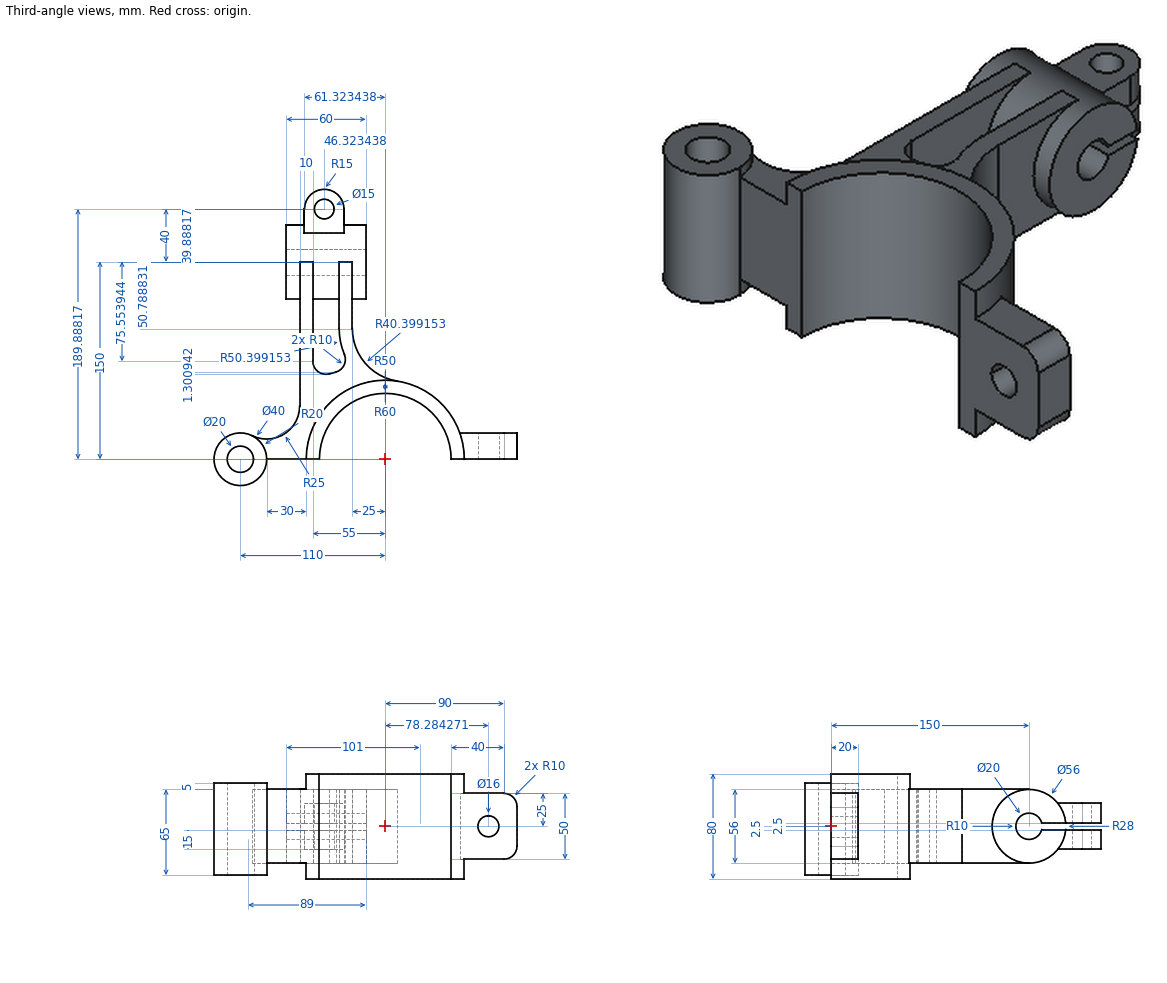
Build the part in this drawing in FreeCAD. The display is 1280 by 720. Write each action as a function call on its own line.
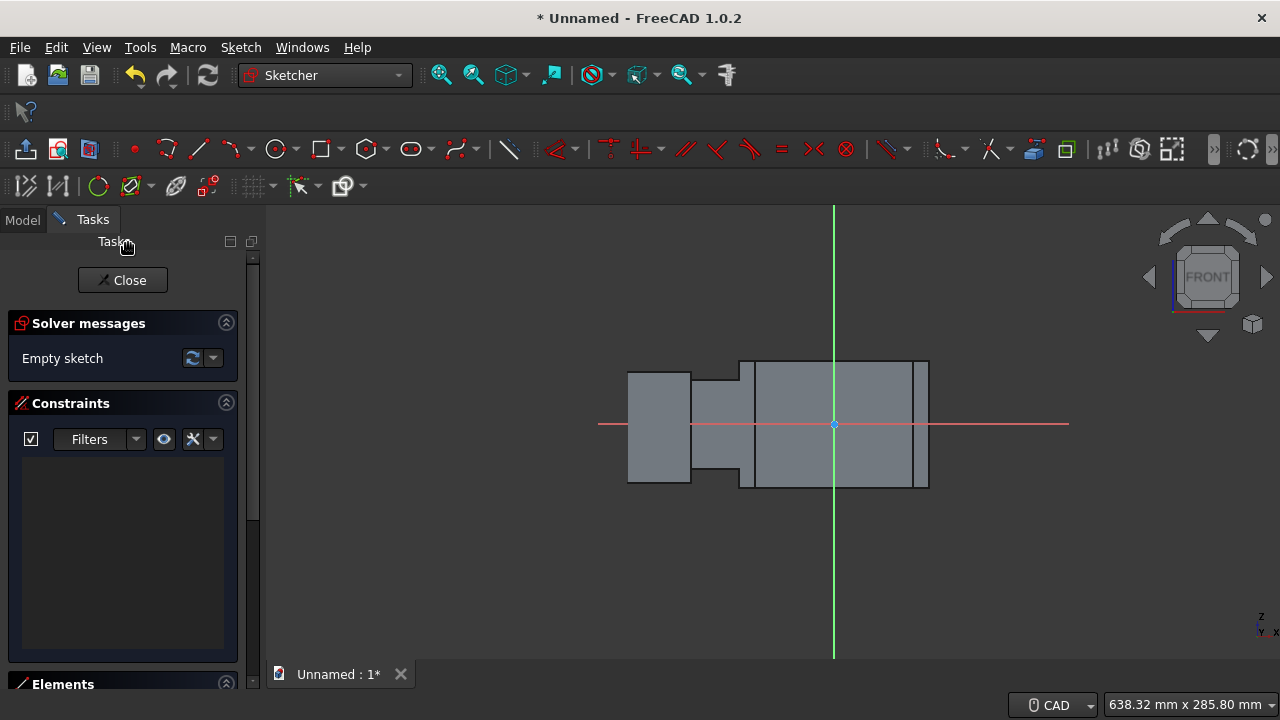
key(q)
key(s)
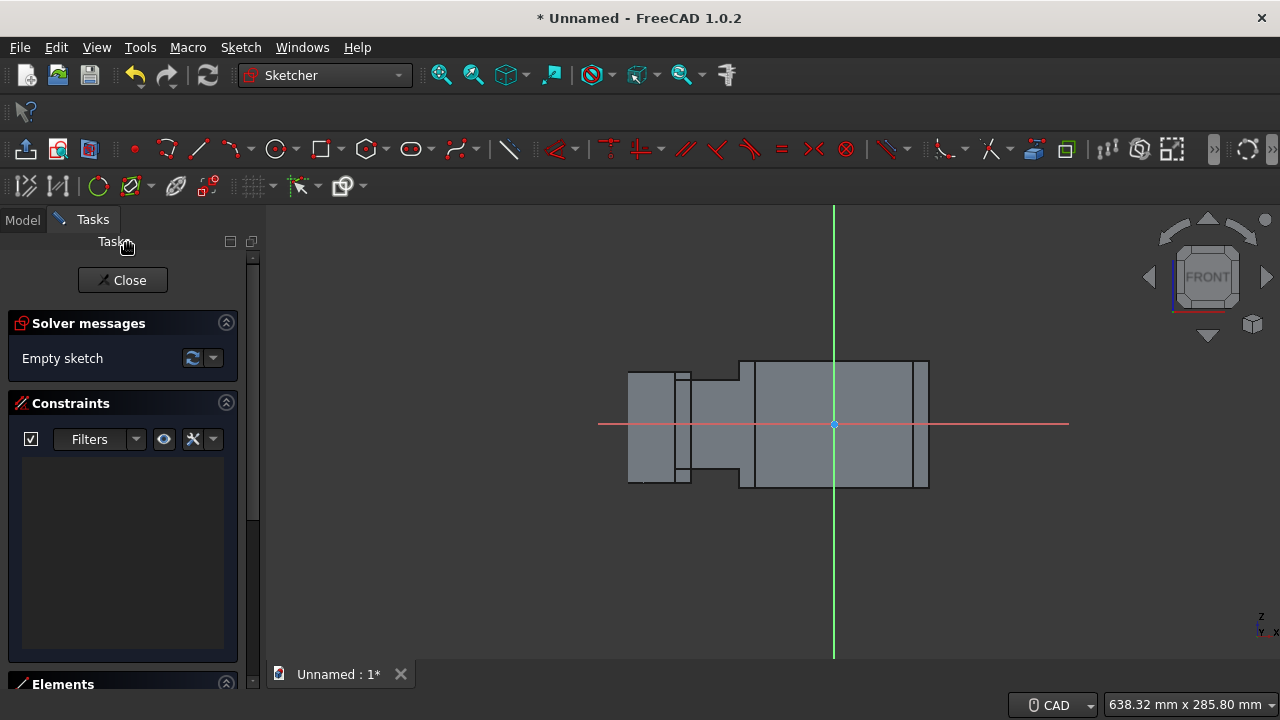
scroll(1004, 421, up, 6)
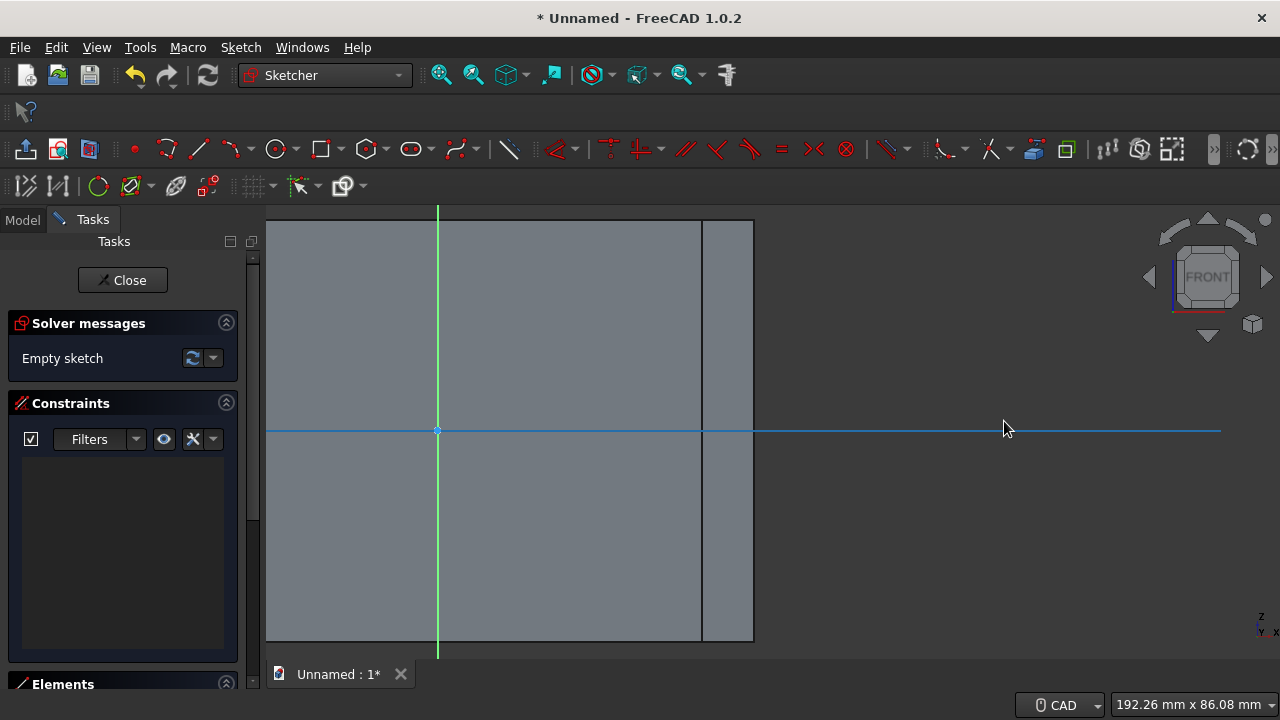
click(168, 150)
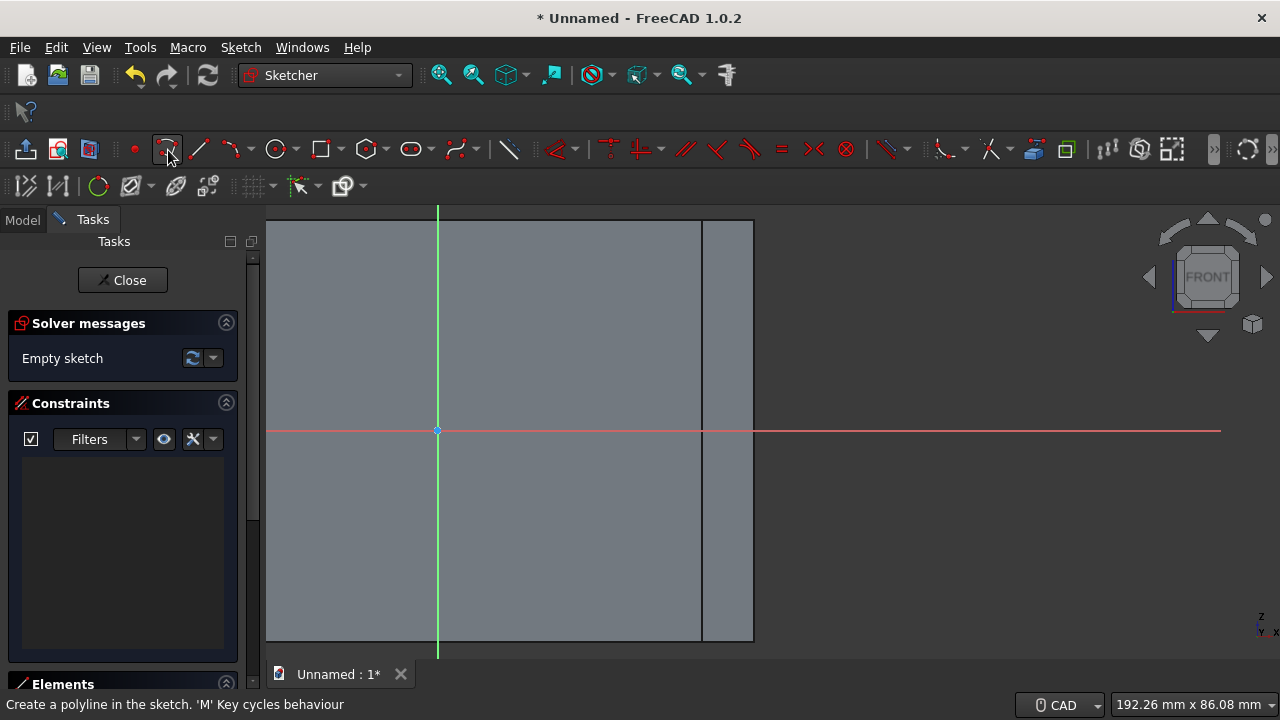
click(913, 299)
click(702, 299)
click(702, 563)
click(913, 563)
right_click(913, 563)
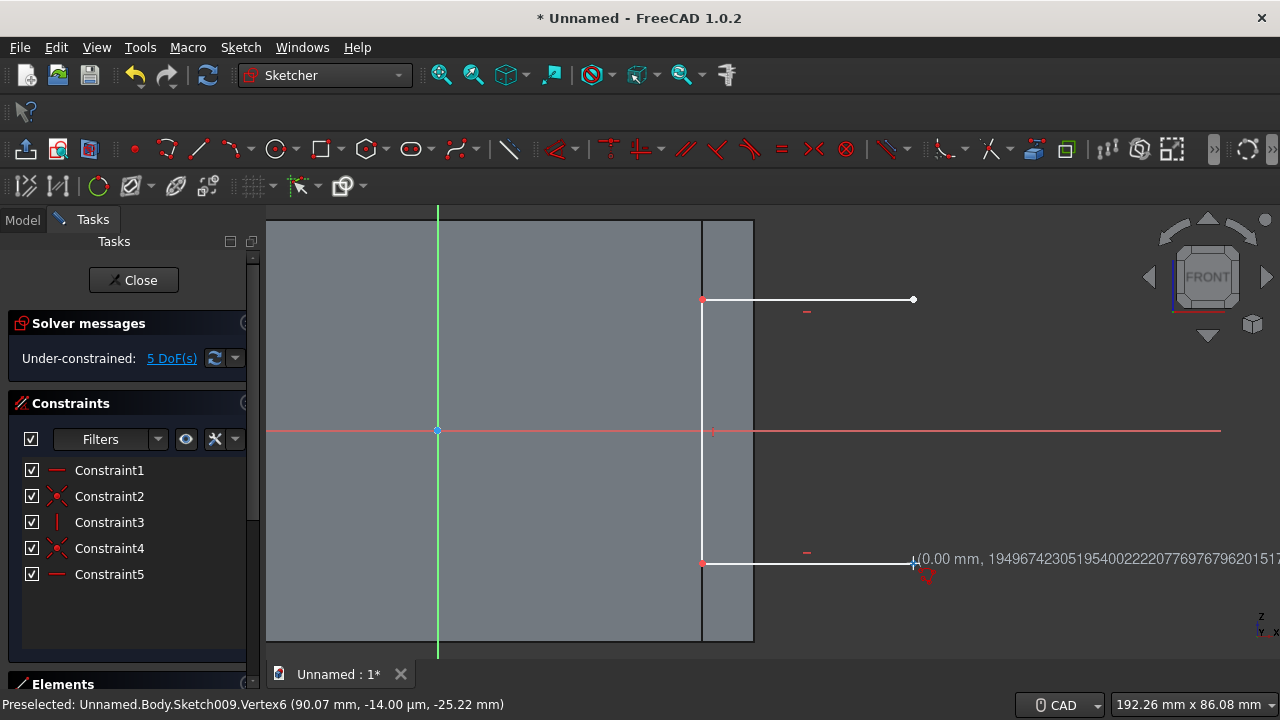
key(g)
key(l)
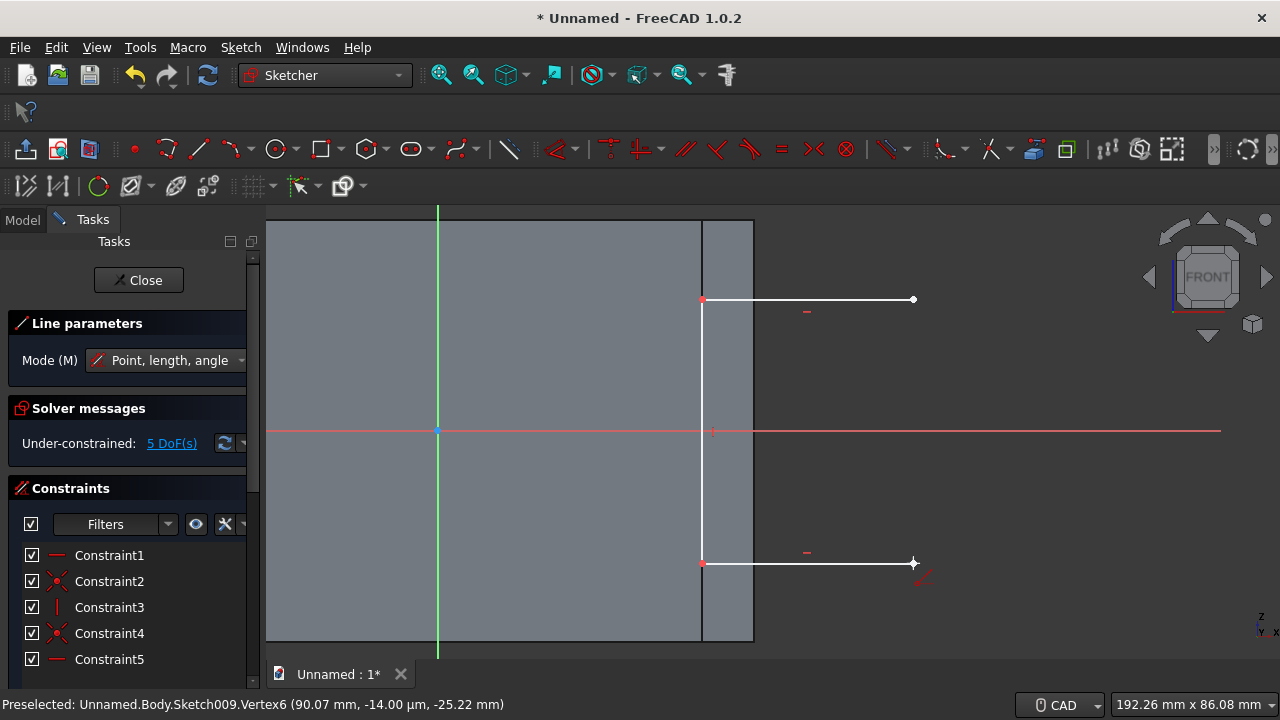
click(965, 510)
click(965, 352)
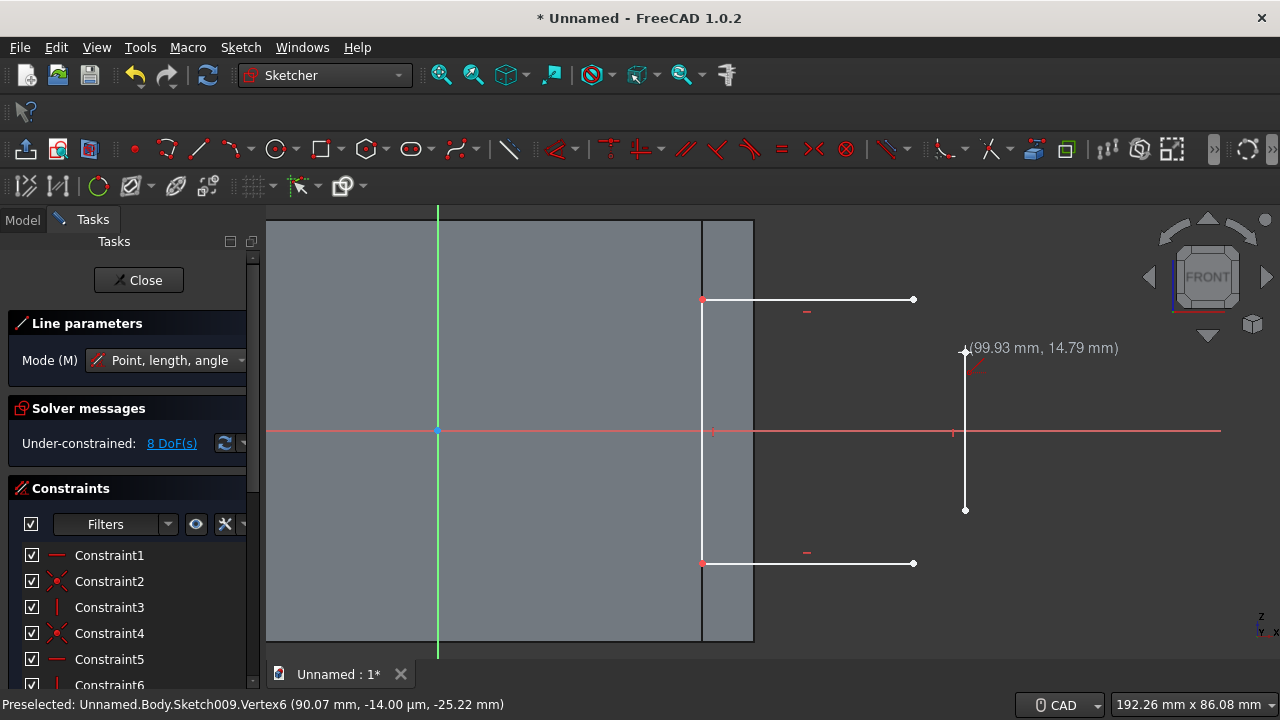
click(232, 150)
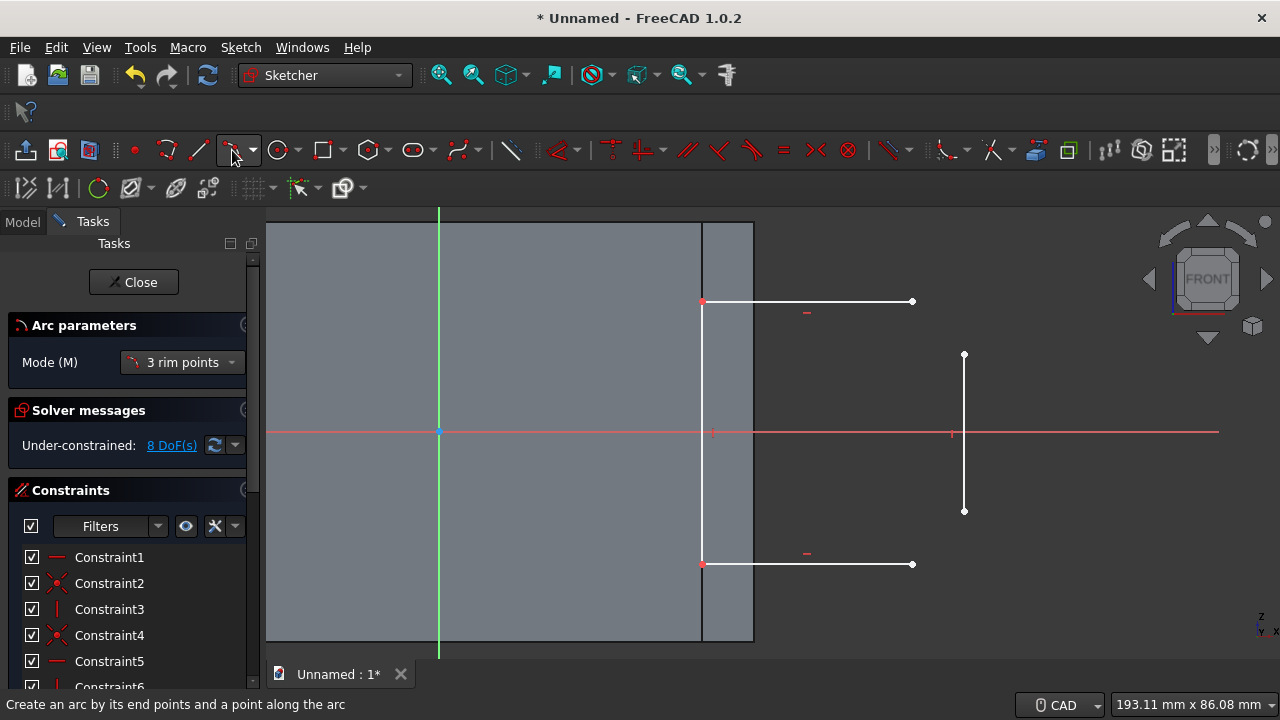
click(912, 564)
click(964, 512)
click(949, 548)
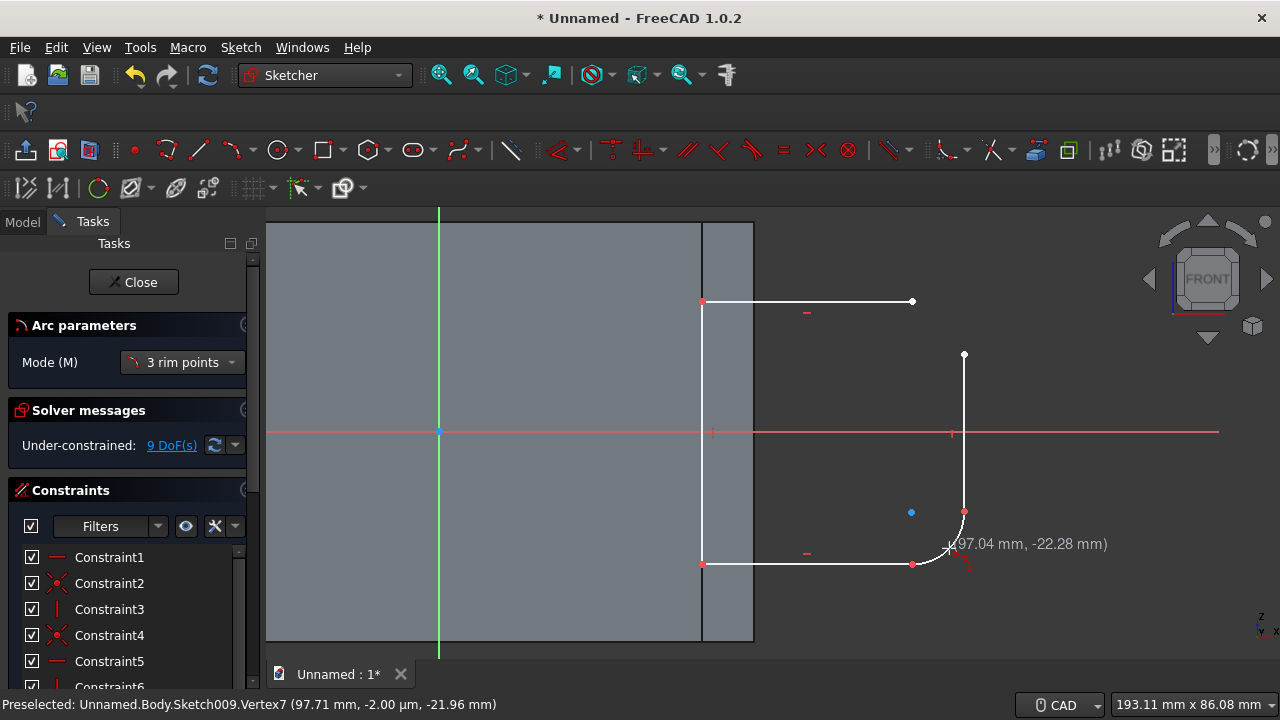
click(964, 354)
click(912, 302)
click(949, 316)
key(Escape)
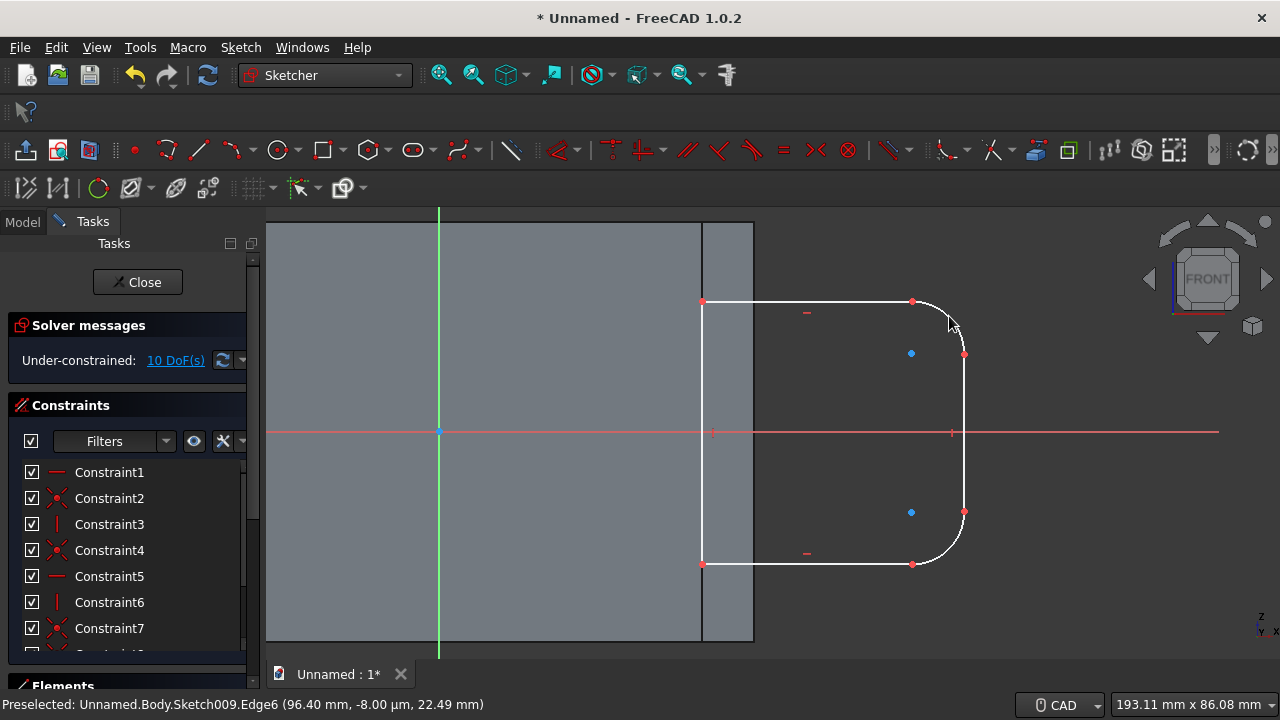
click(849, 302)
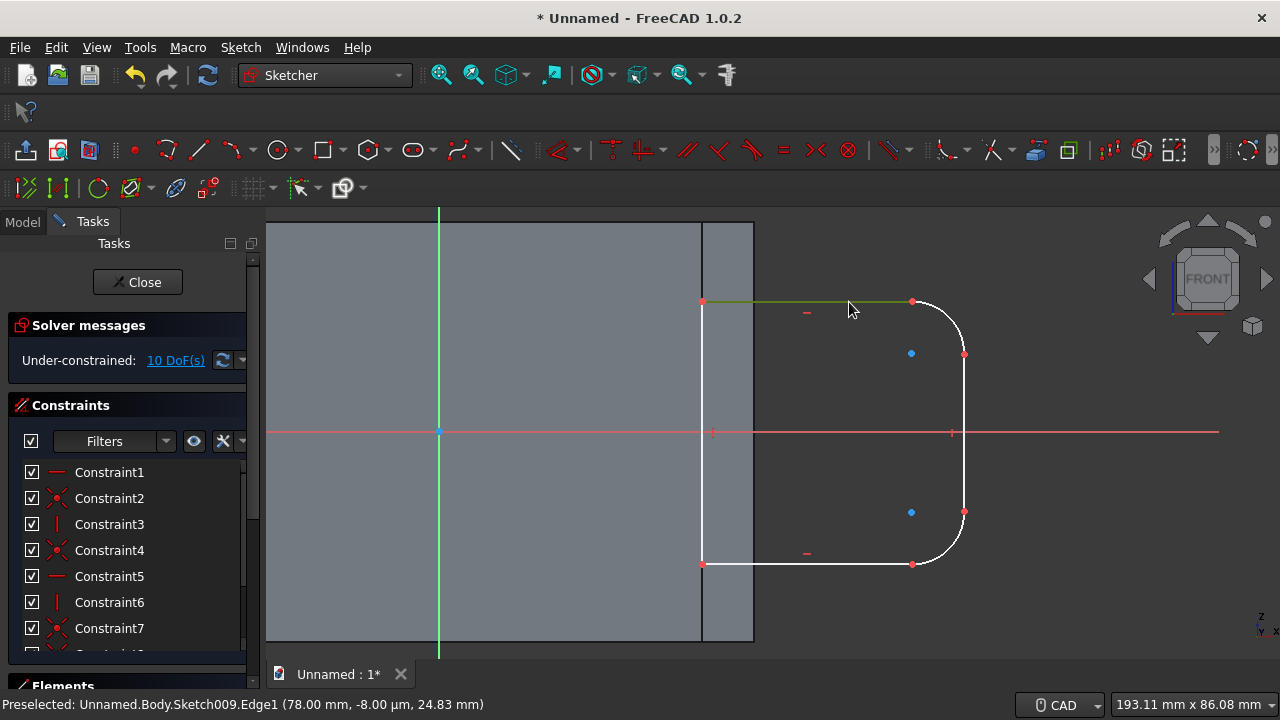
click(959, 331)